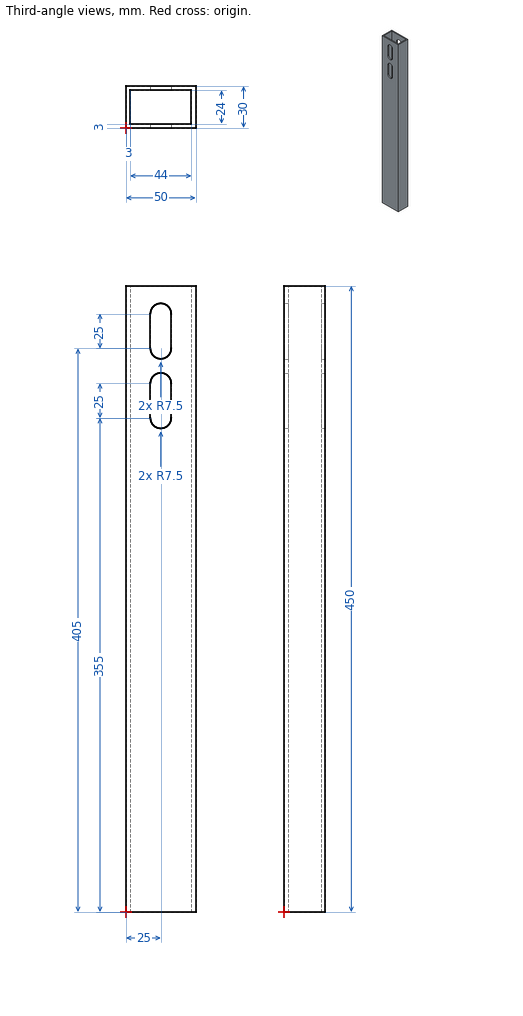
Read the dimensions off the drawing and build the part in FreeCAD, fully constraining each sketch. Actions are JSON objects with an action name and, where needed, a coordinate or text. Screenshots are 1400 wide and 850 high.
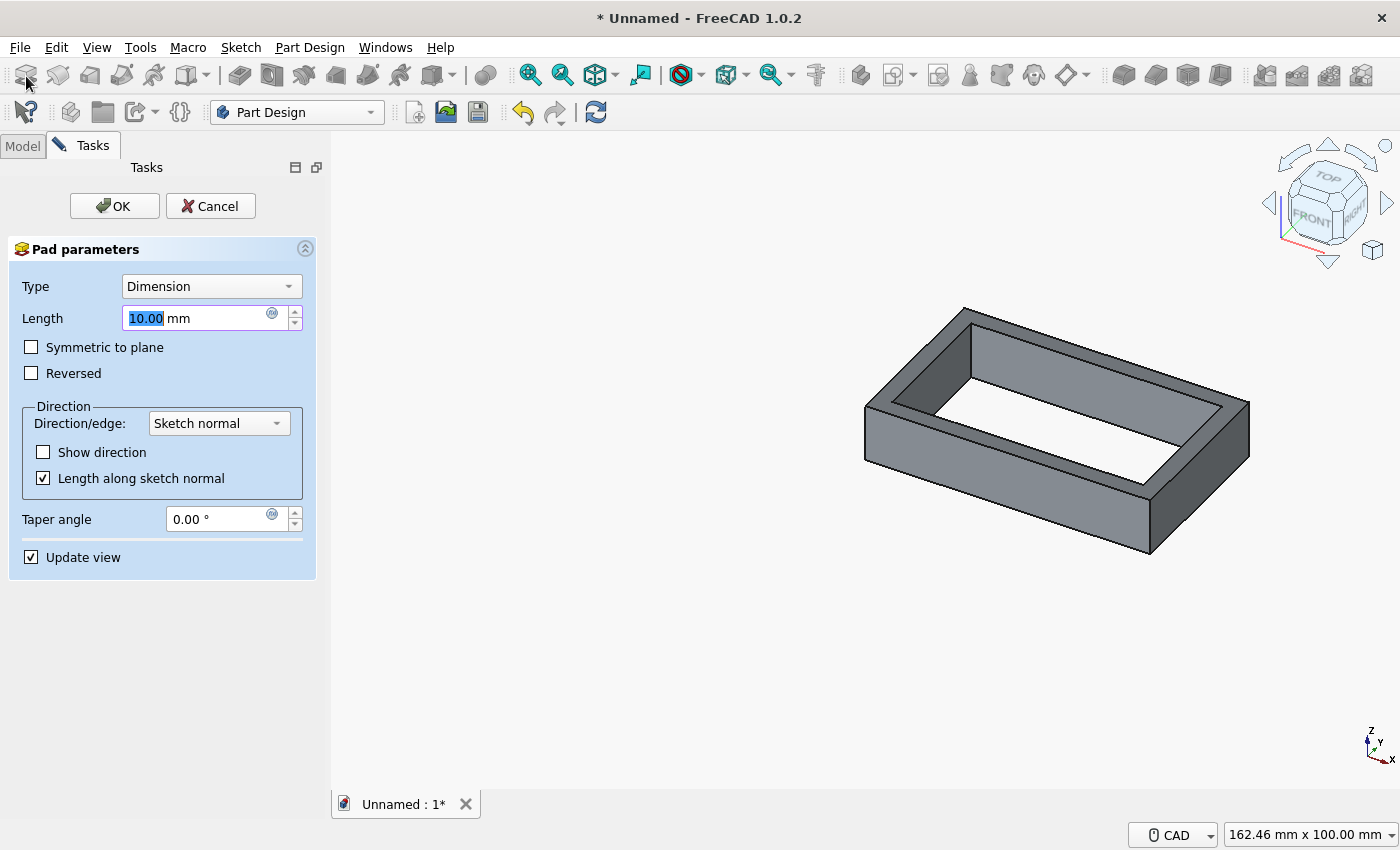
{"action": "type", "text": "450"}
{"action": "key", "text": "Tab"}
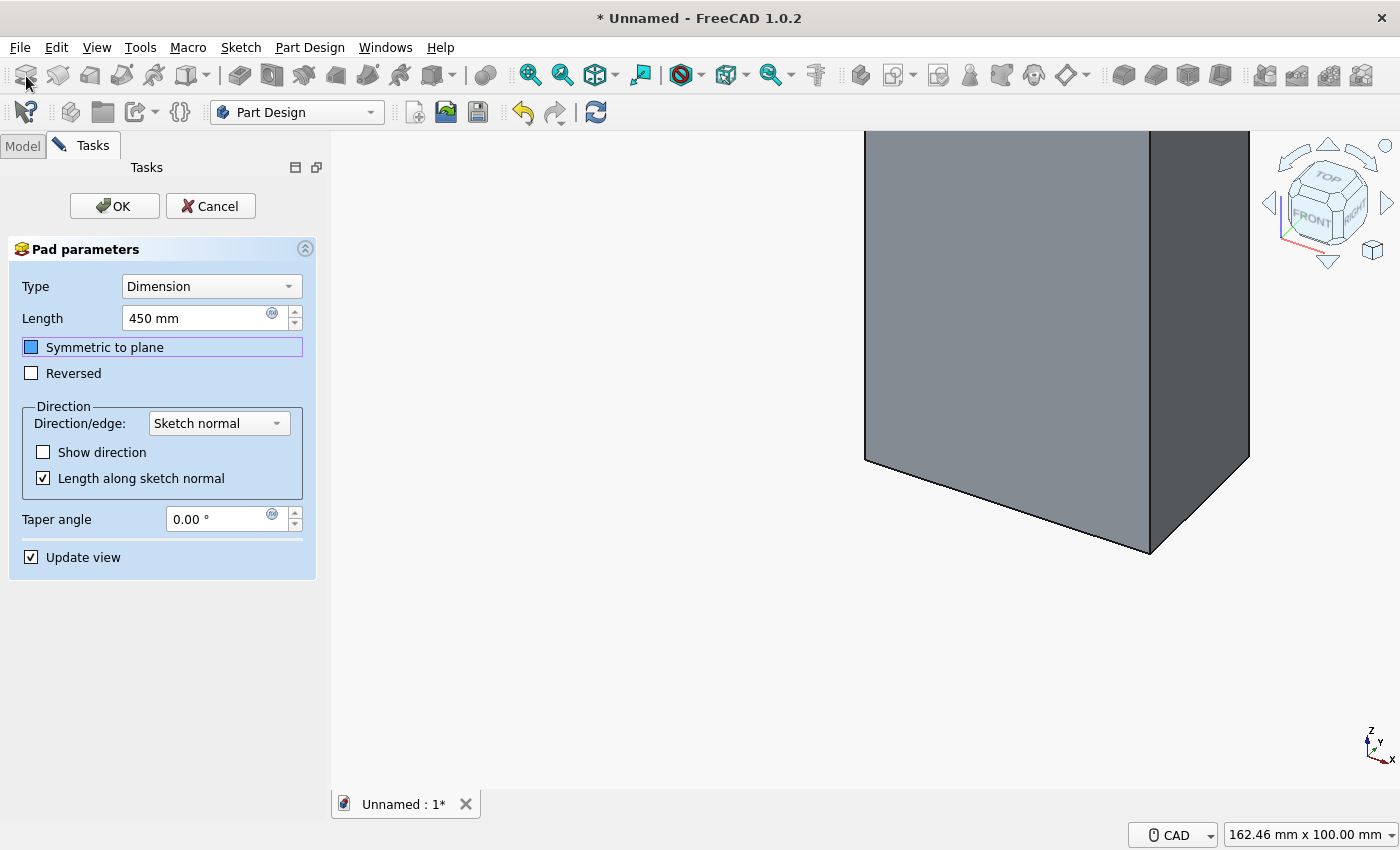
{"action": "left_click", "coordinate": [115, 206]}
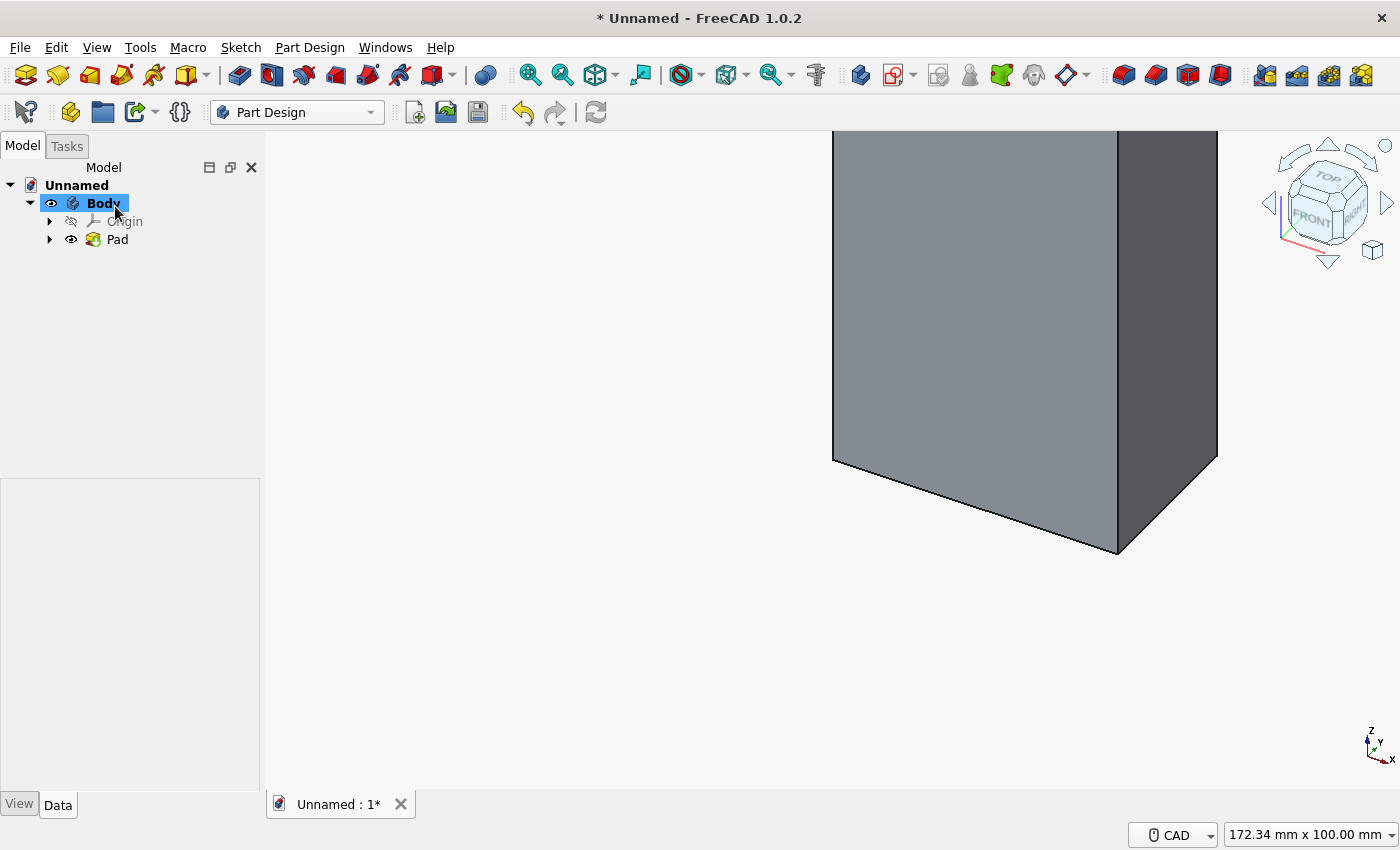
{"action": "left_click", "coordinate": [532, 76]}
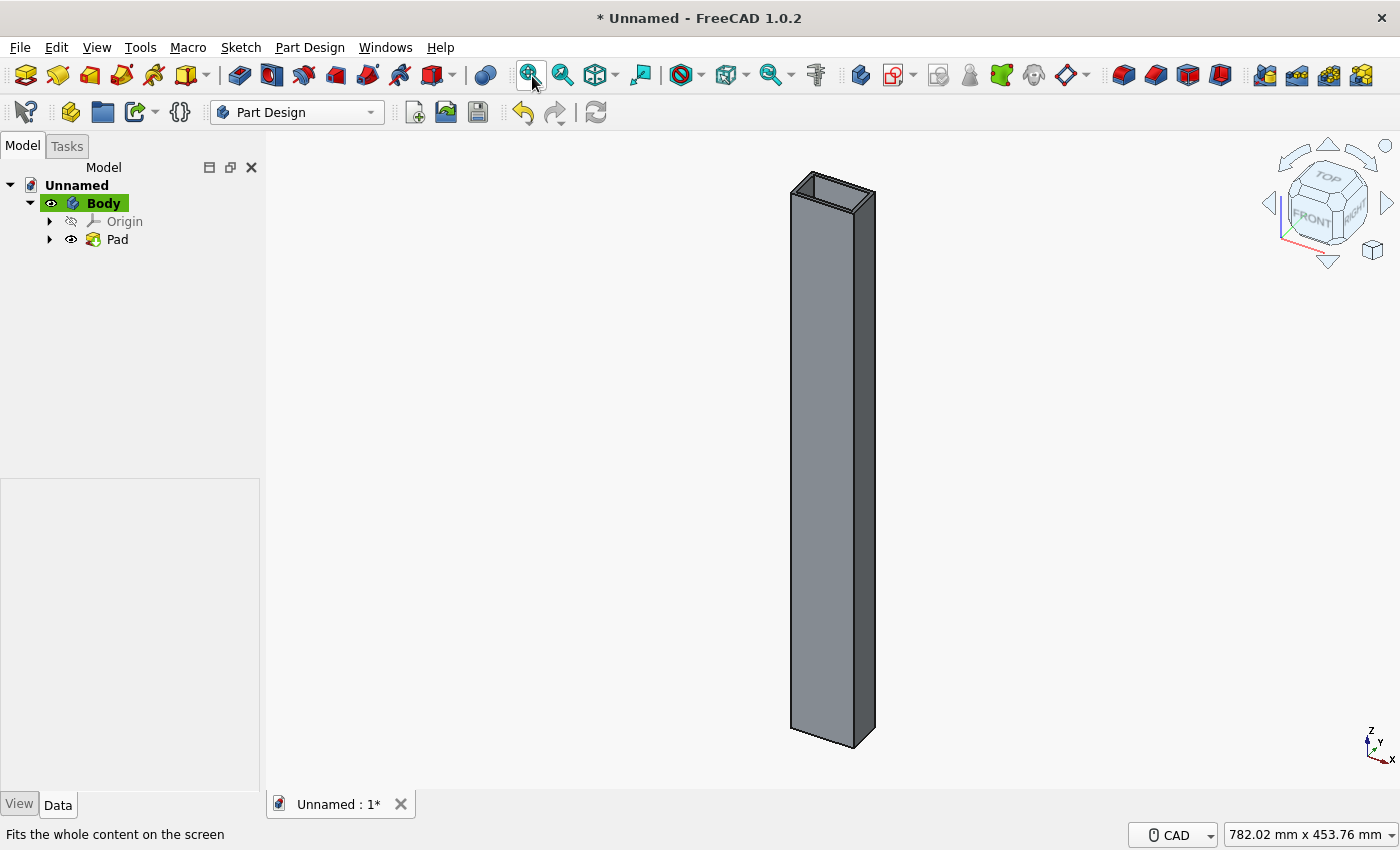
{"action": "left_click", "coordinate": [894, 76]}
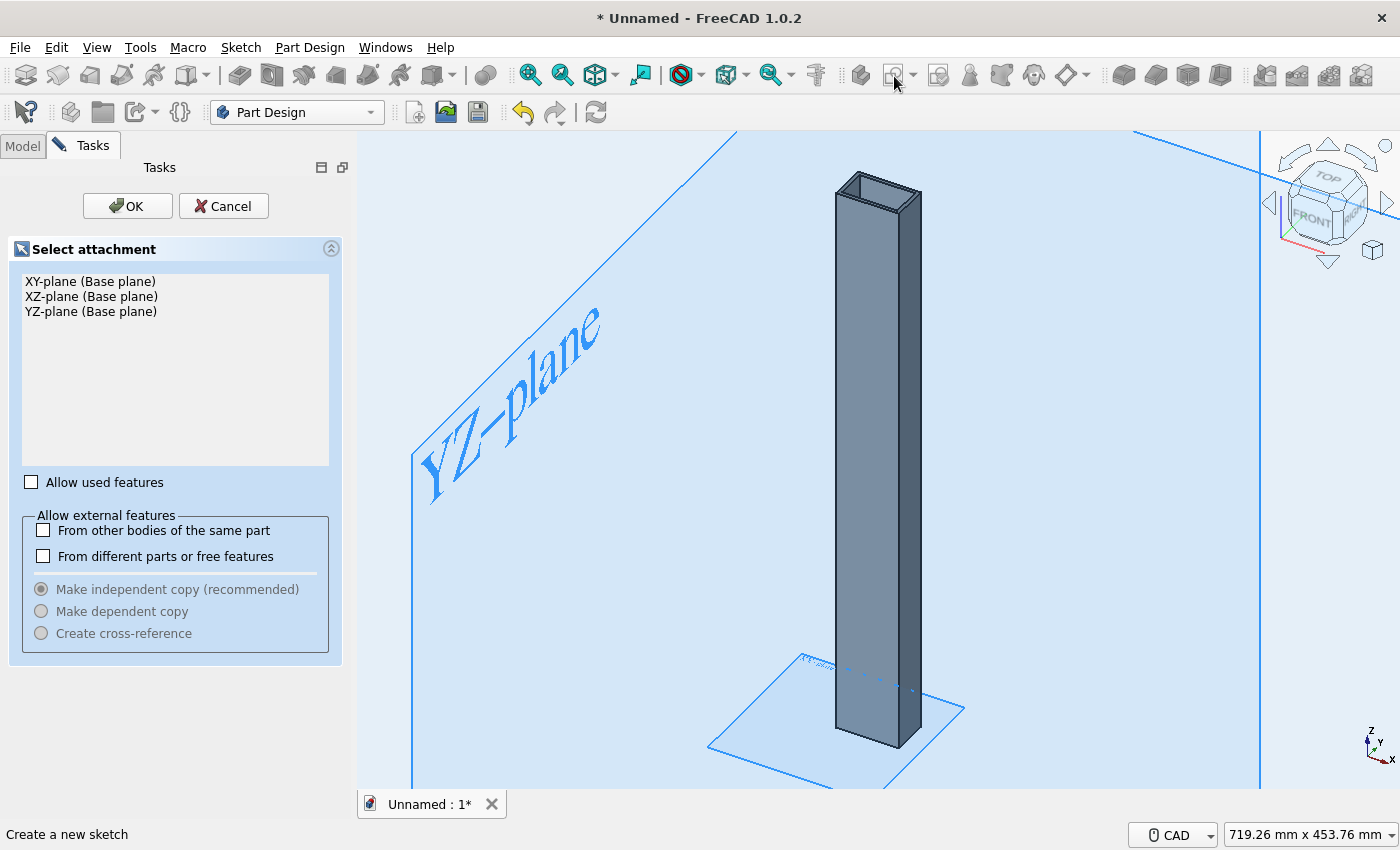
{"action": "left_click", "coordinate": [82, 296]}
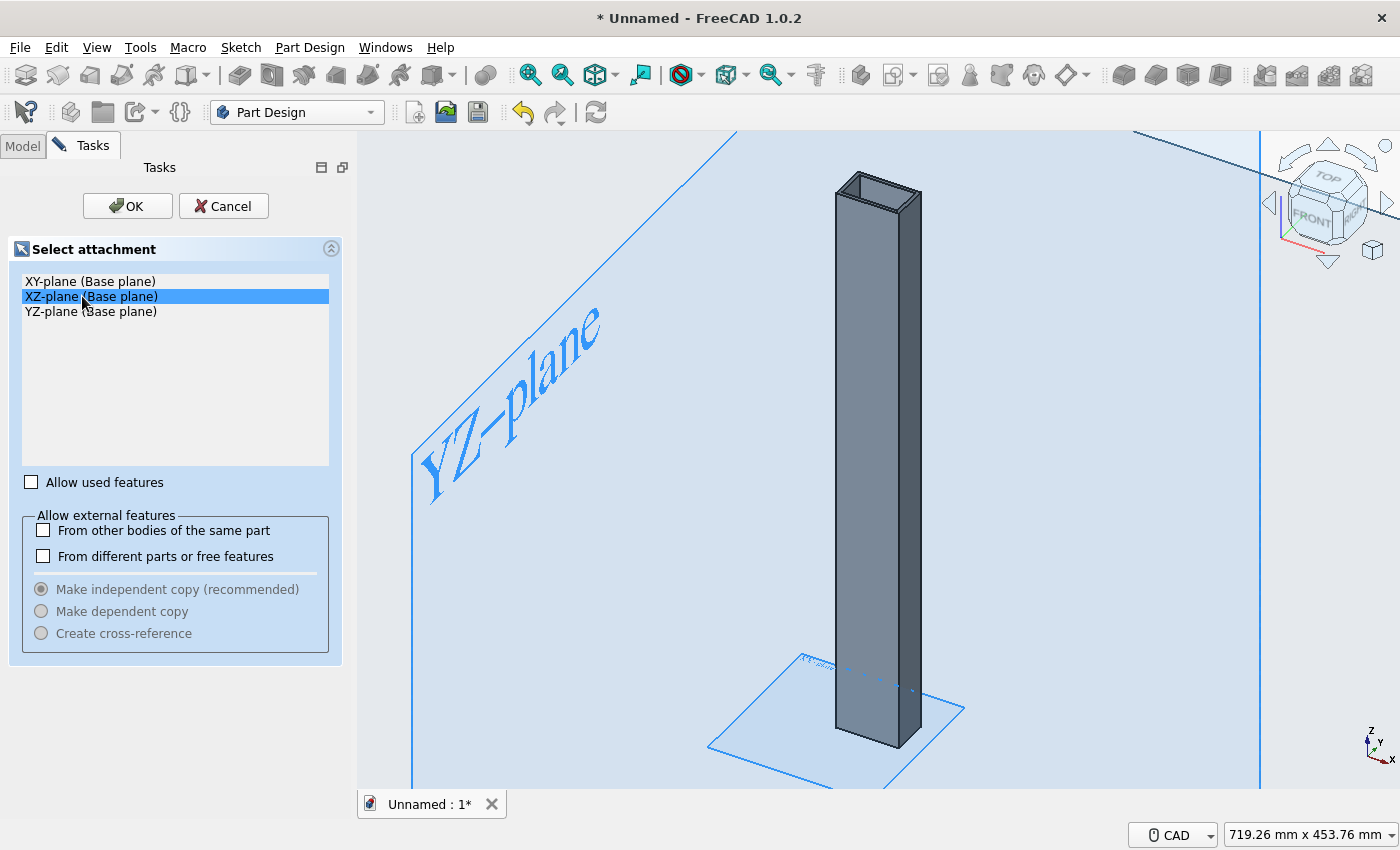
{"action": "left_click", "coordinate": [128, 206]}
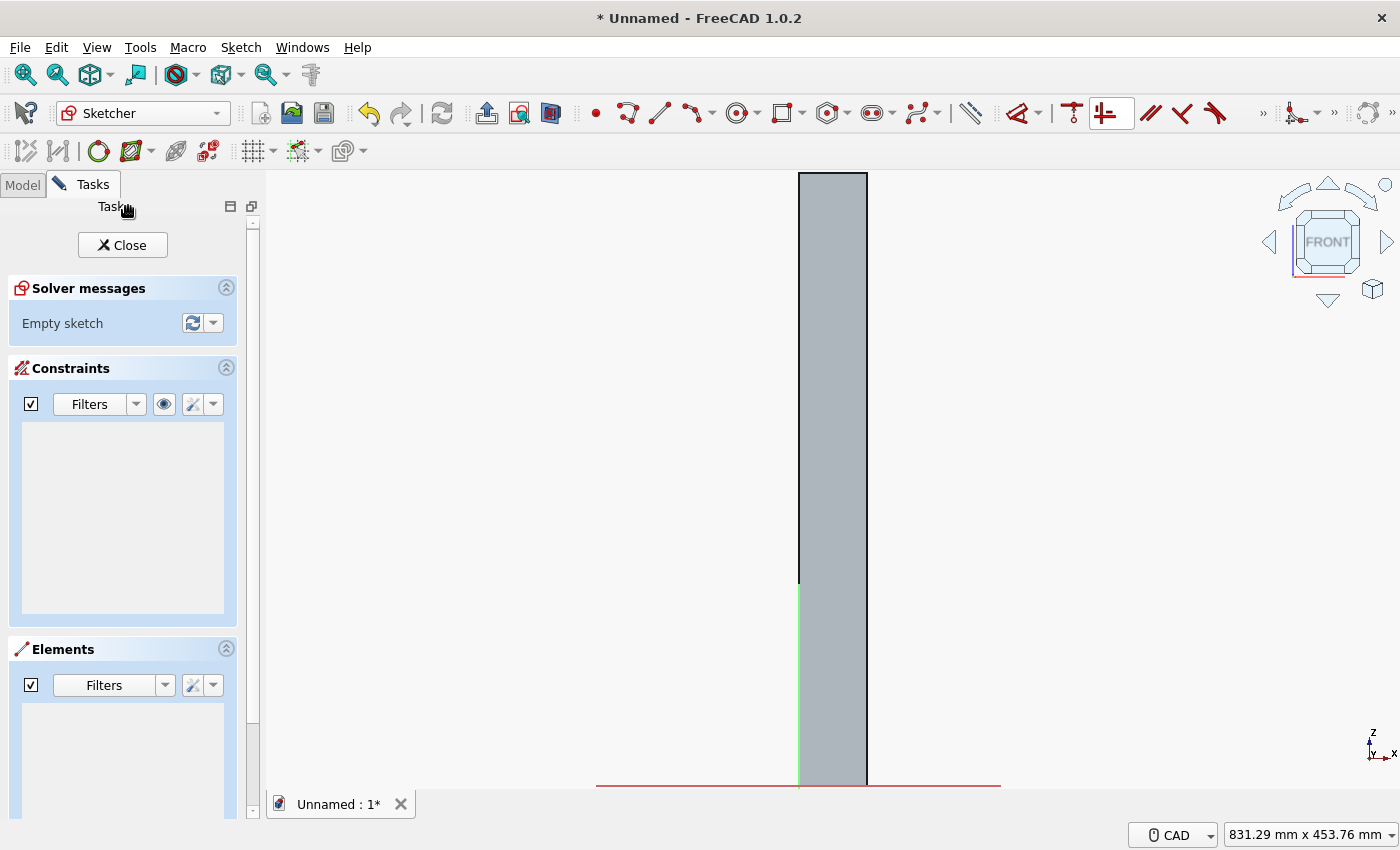
{"action": "scroll", "coordinate": [764, 480], "scroll_direction": "down", "scroll_amount": 5}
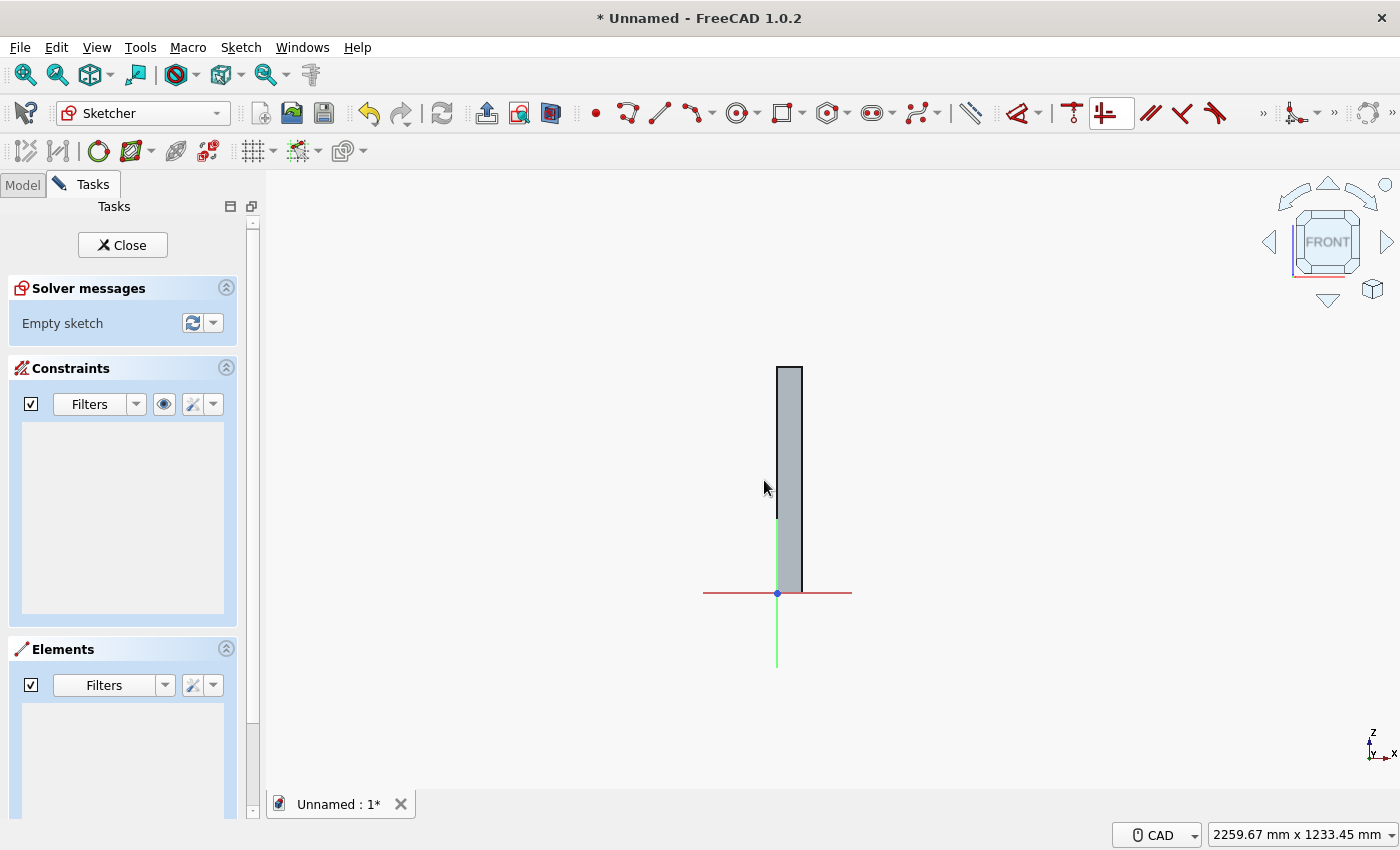
{"action": "scroll", "coordinate": [791, 378], "scroll_direction": "up", "scroll_amount": 15}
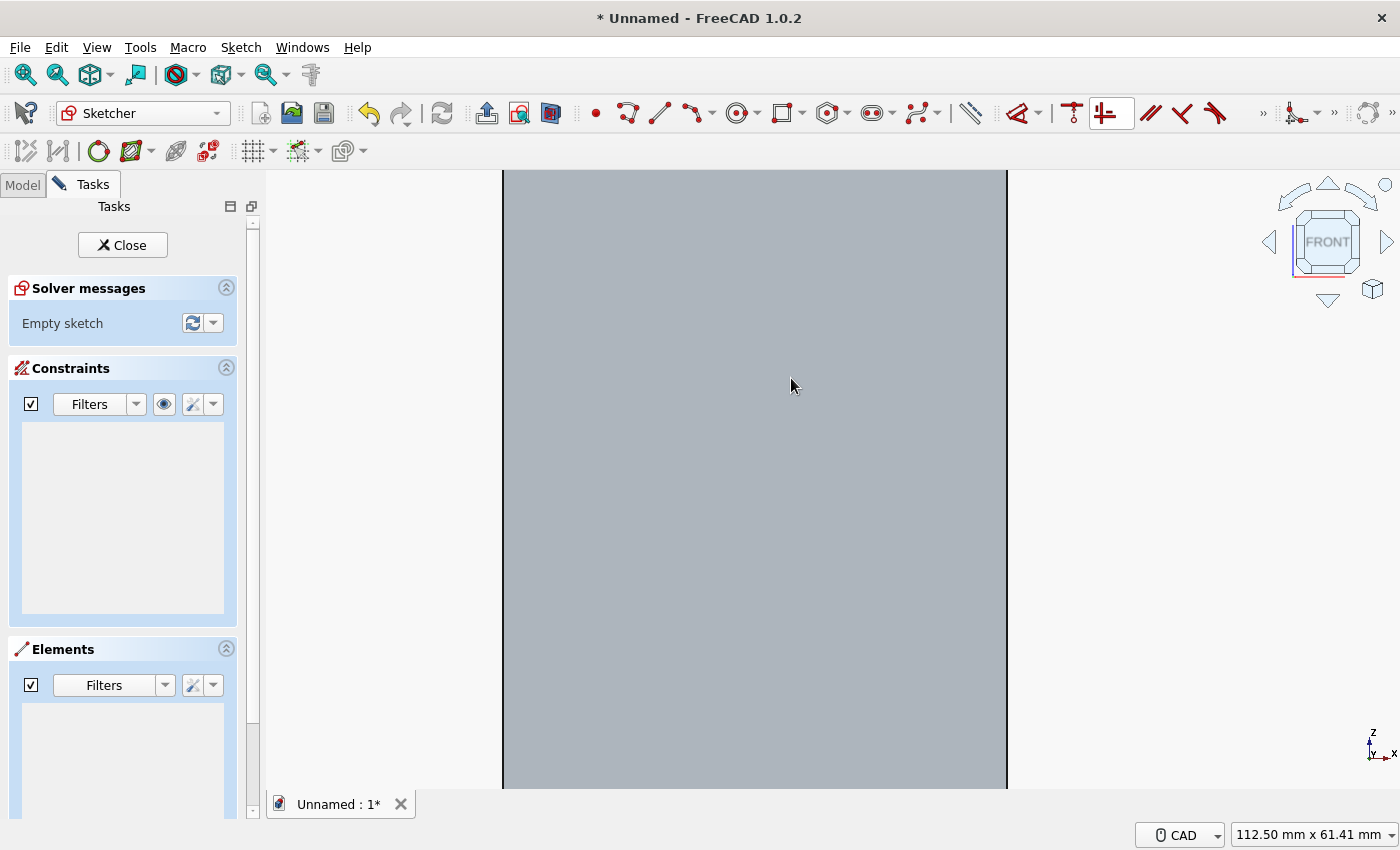
{"action": "key", "text": "g s"}